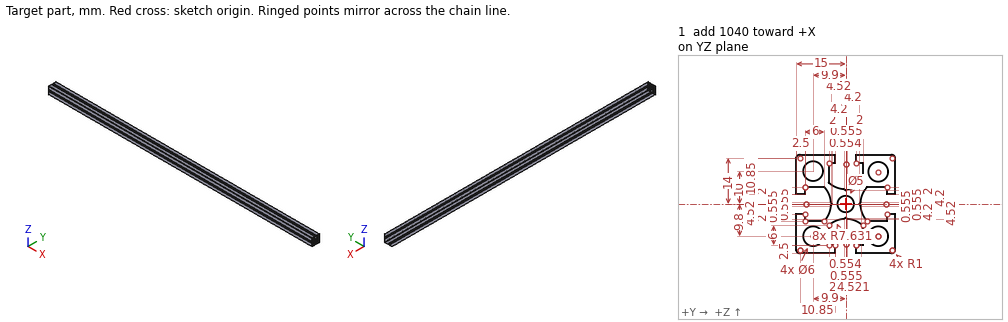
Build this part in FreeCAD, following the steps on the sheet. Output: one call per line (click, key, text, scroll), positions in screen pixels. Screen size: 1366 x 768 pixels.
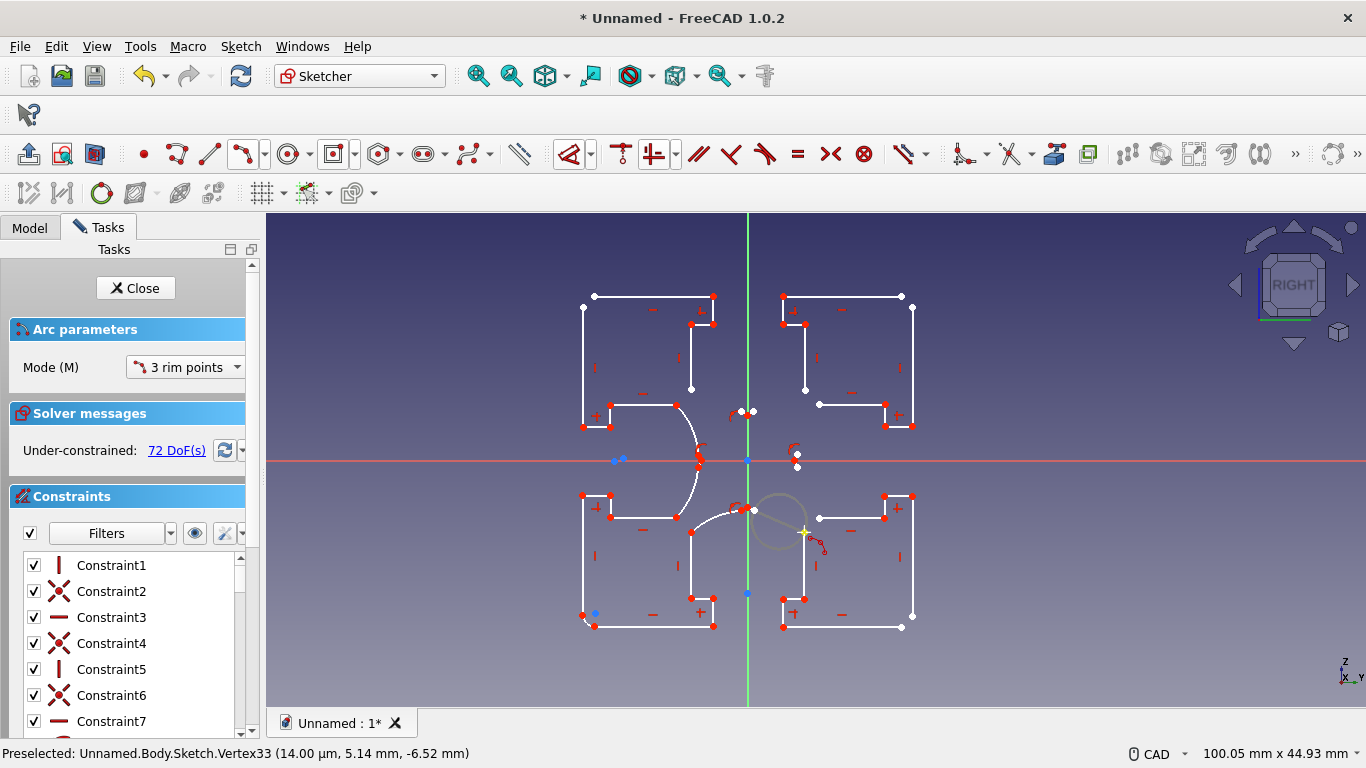
scroll(781, 517, up, 7)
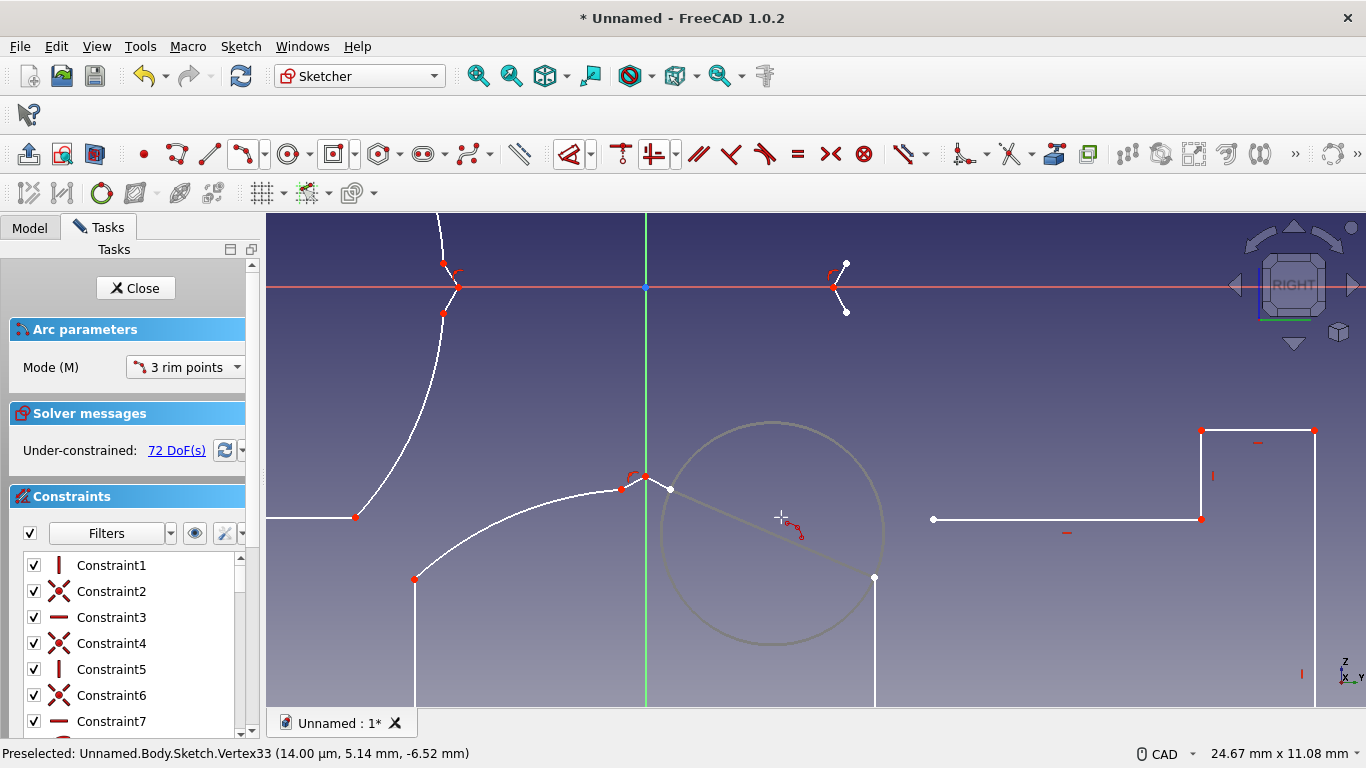
click(780, 515)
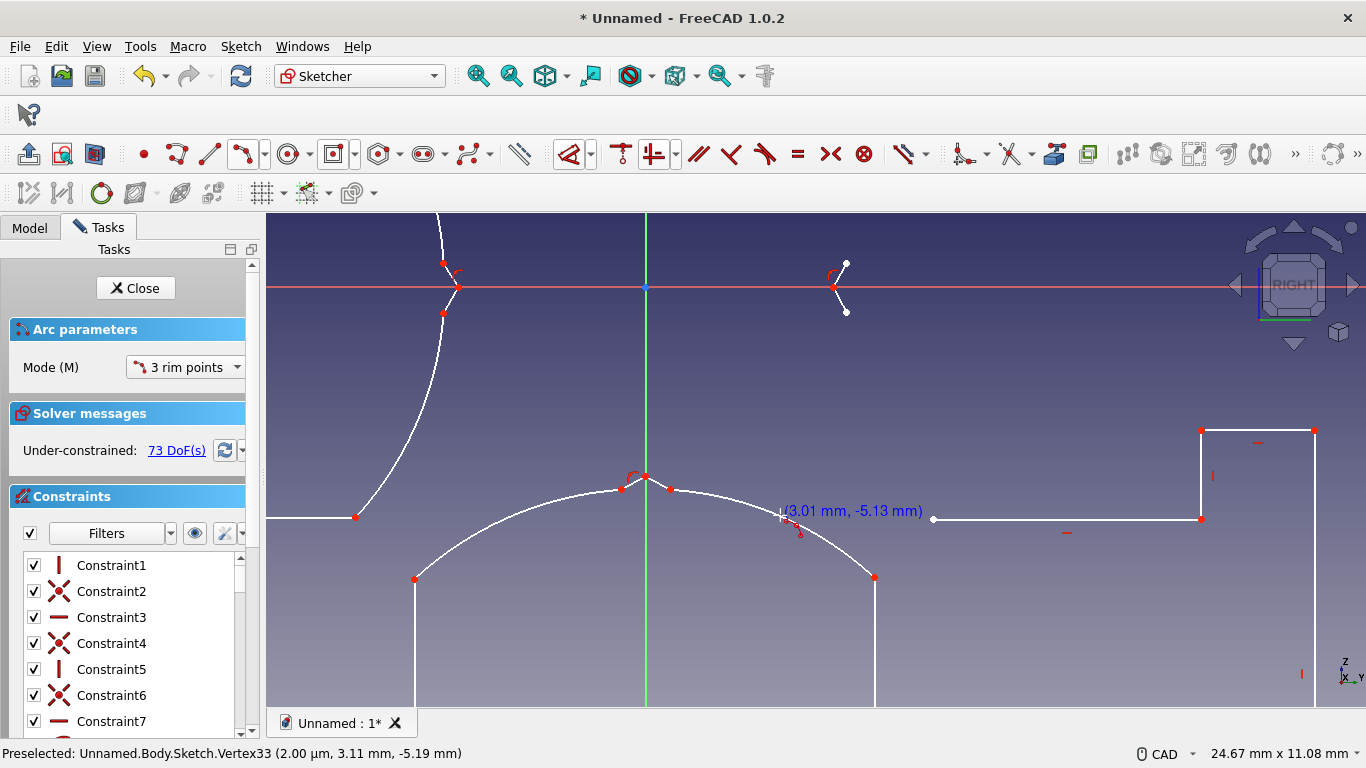
scroll(781, 517, down, 7)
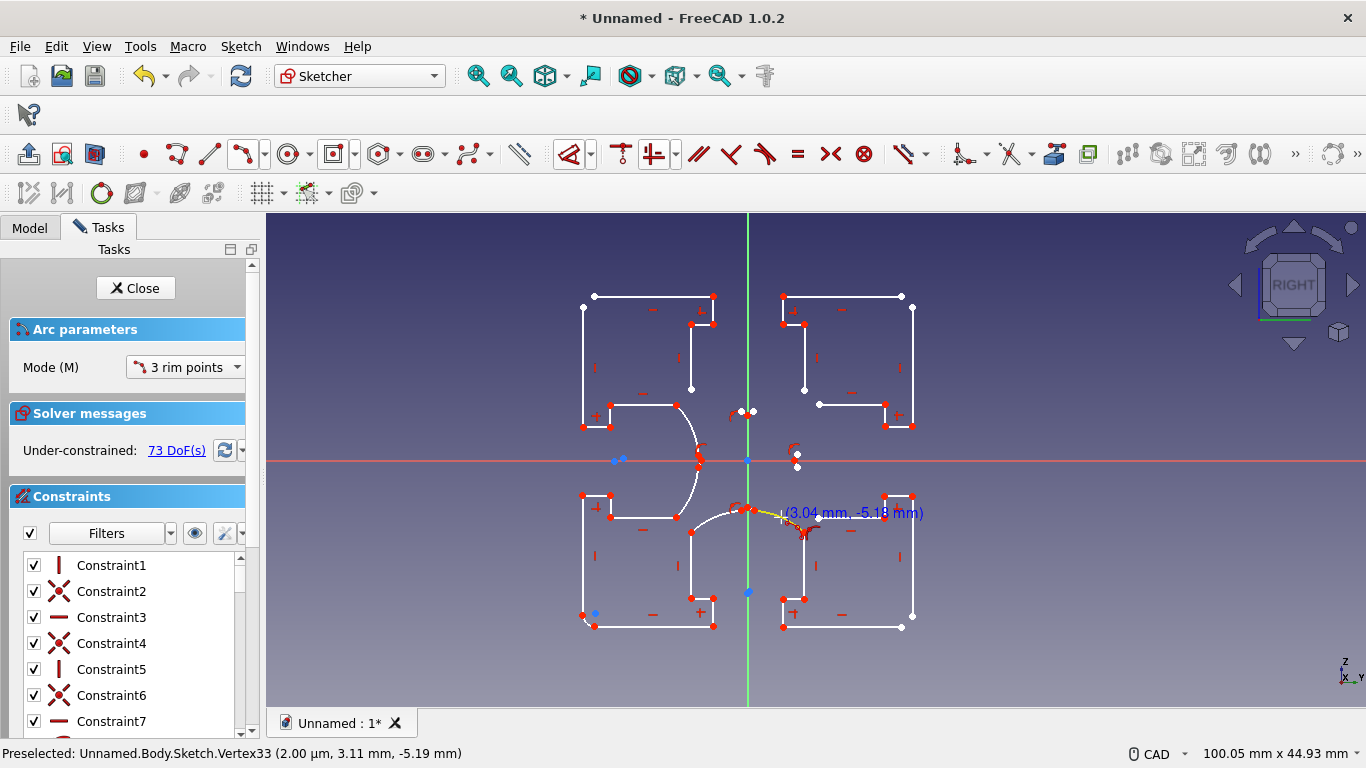
click(902, 627)
click(913, 616)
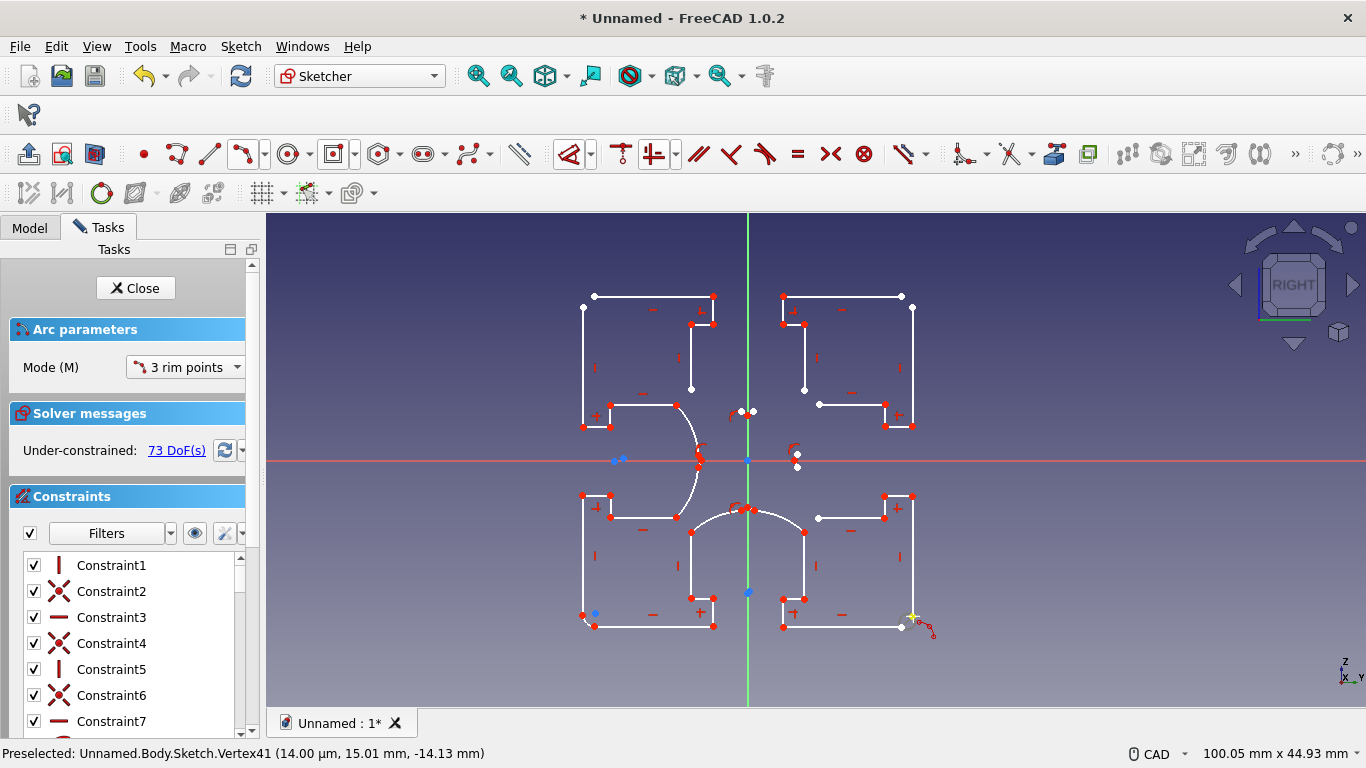
scroll(910, 622, up, 8)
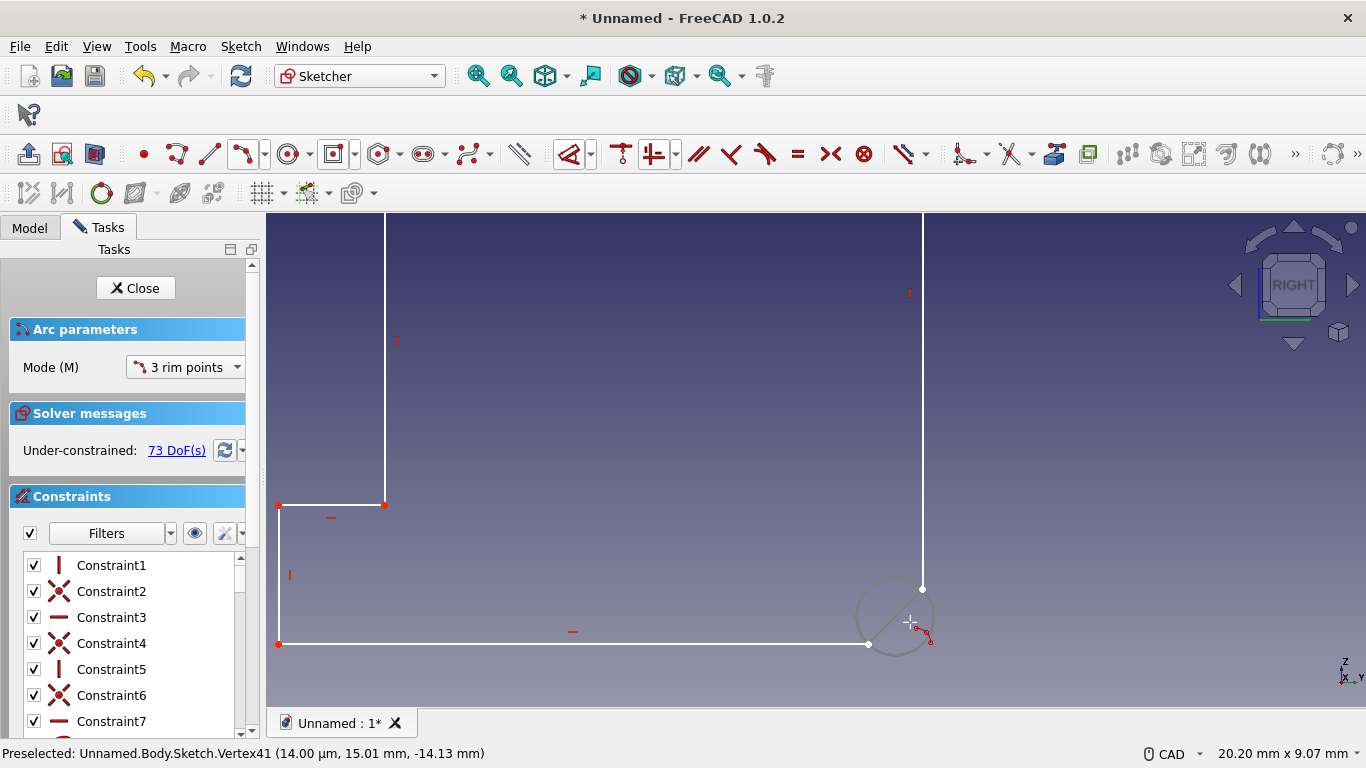
click(906, 621)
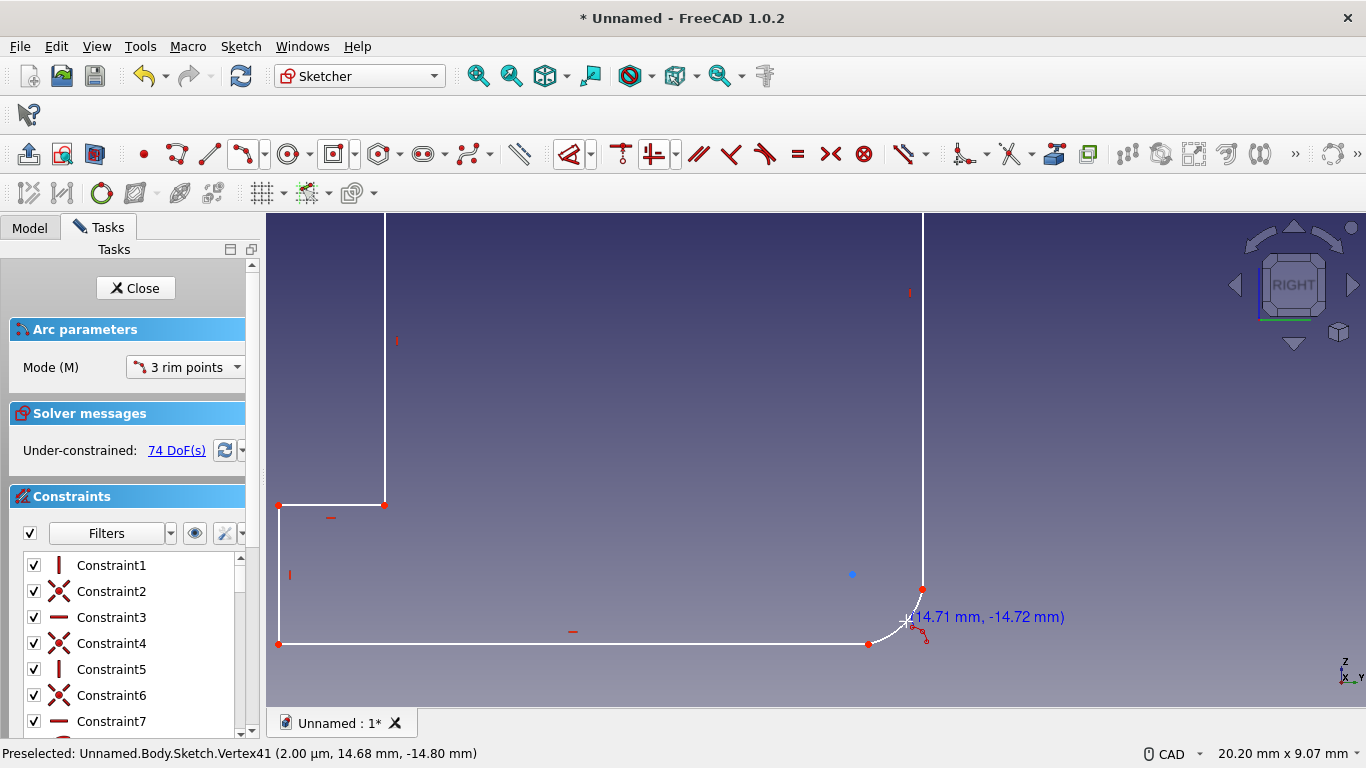
scroll(910, 622, down, 8)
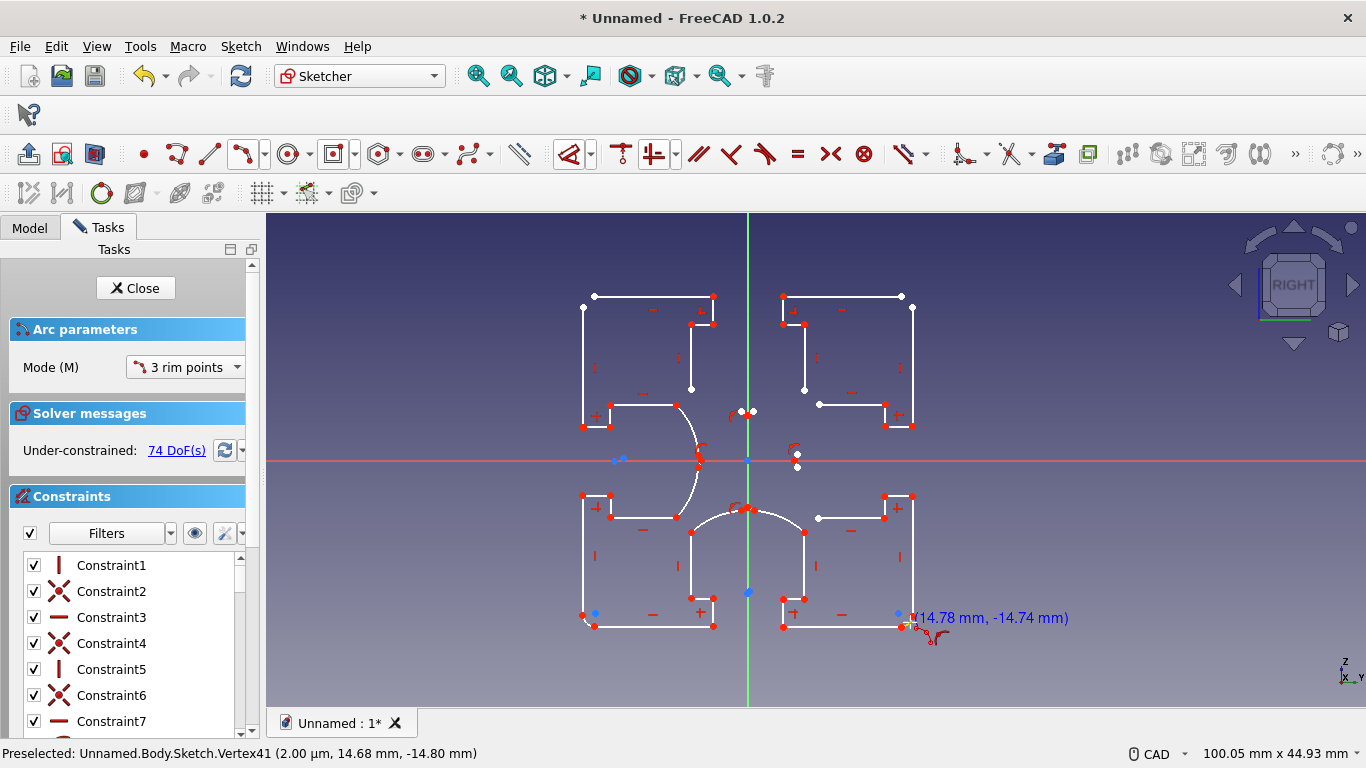
click(819, 518)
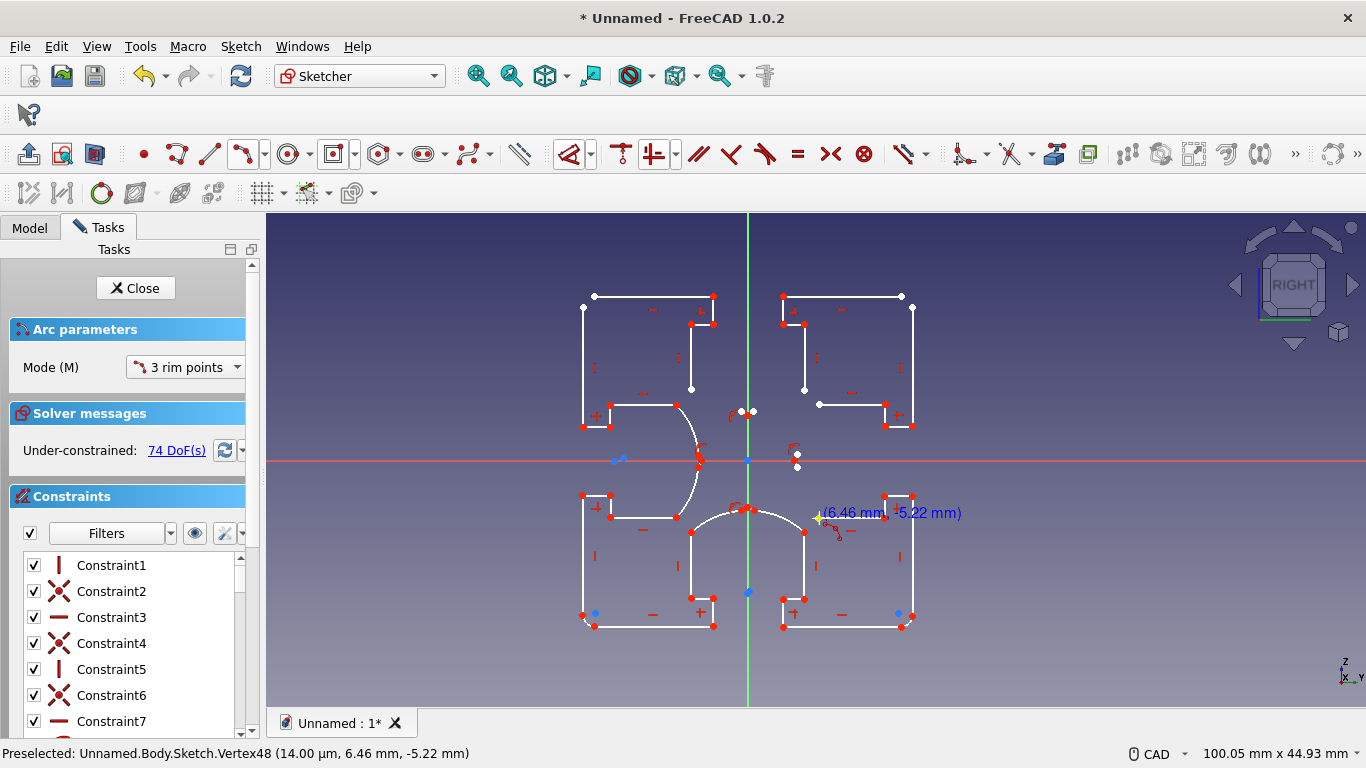
scroll(798, 467, up, 8)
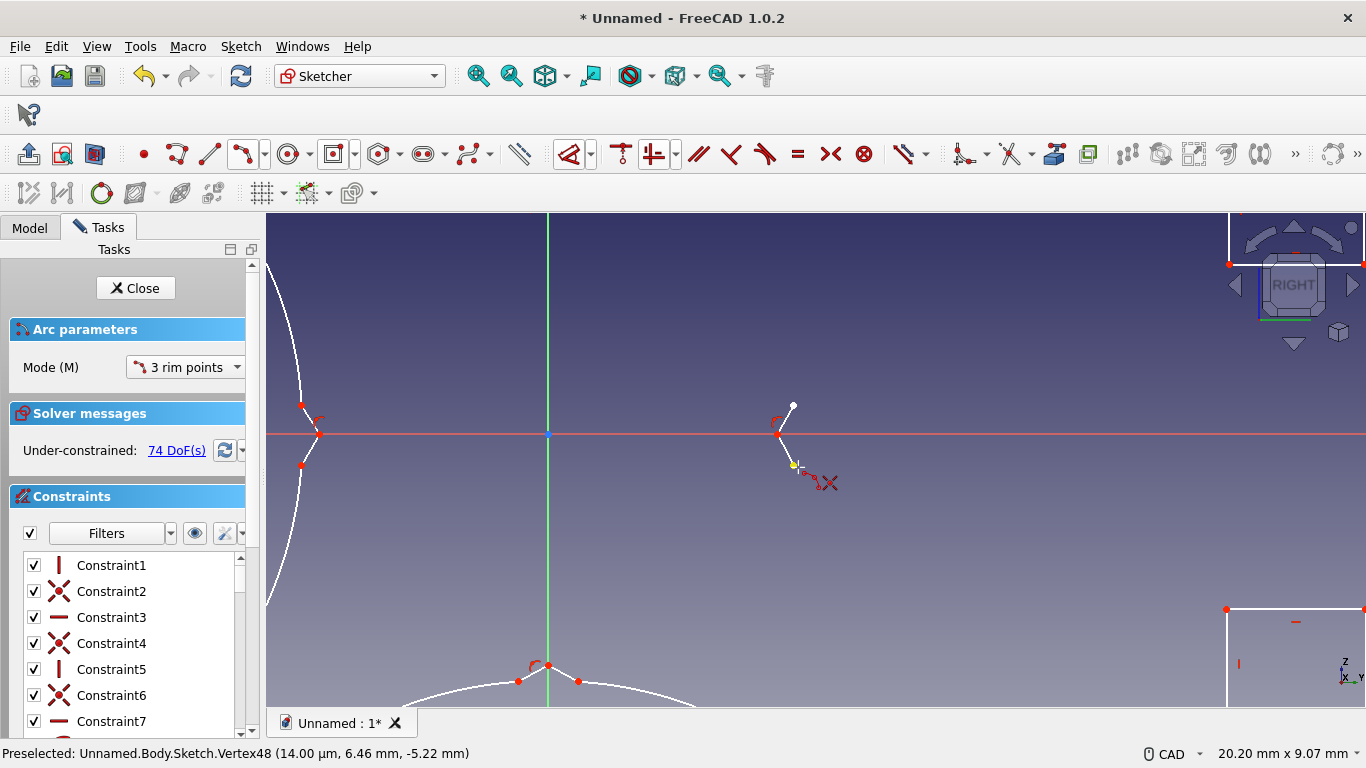
click(794, 465)
click(827, 599)